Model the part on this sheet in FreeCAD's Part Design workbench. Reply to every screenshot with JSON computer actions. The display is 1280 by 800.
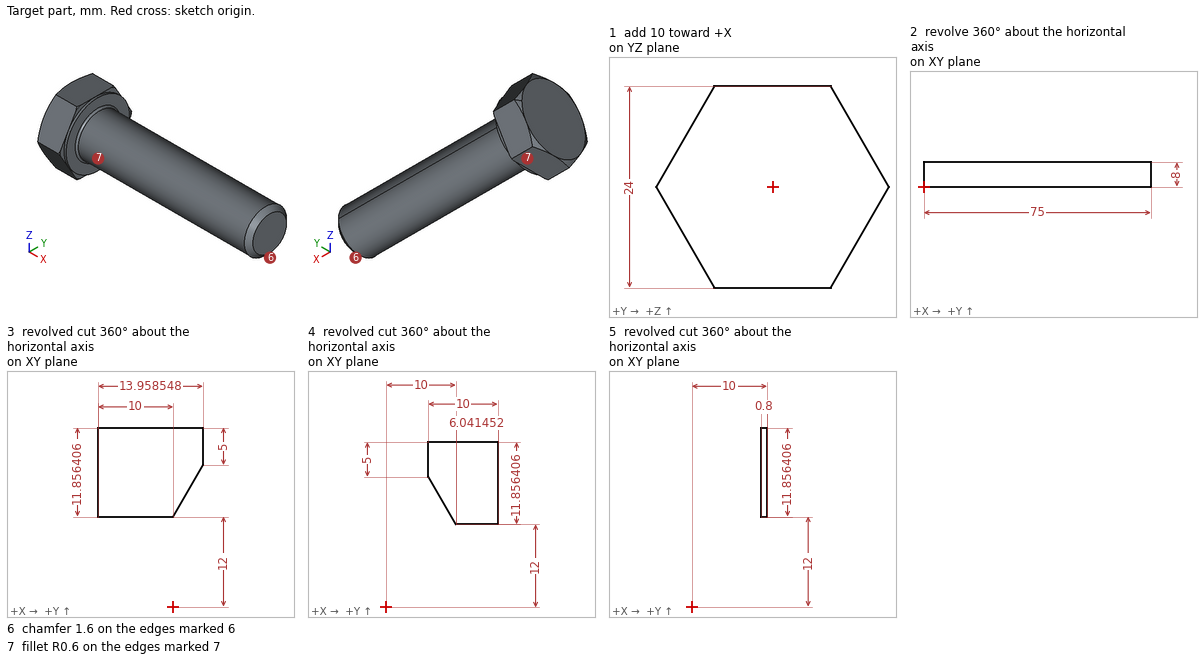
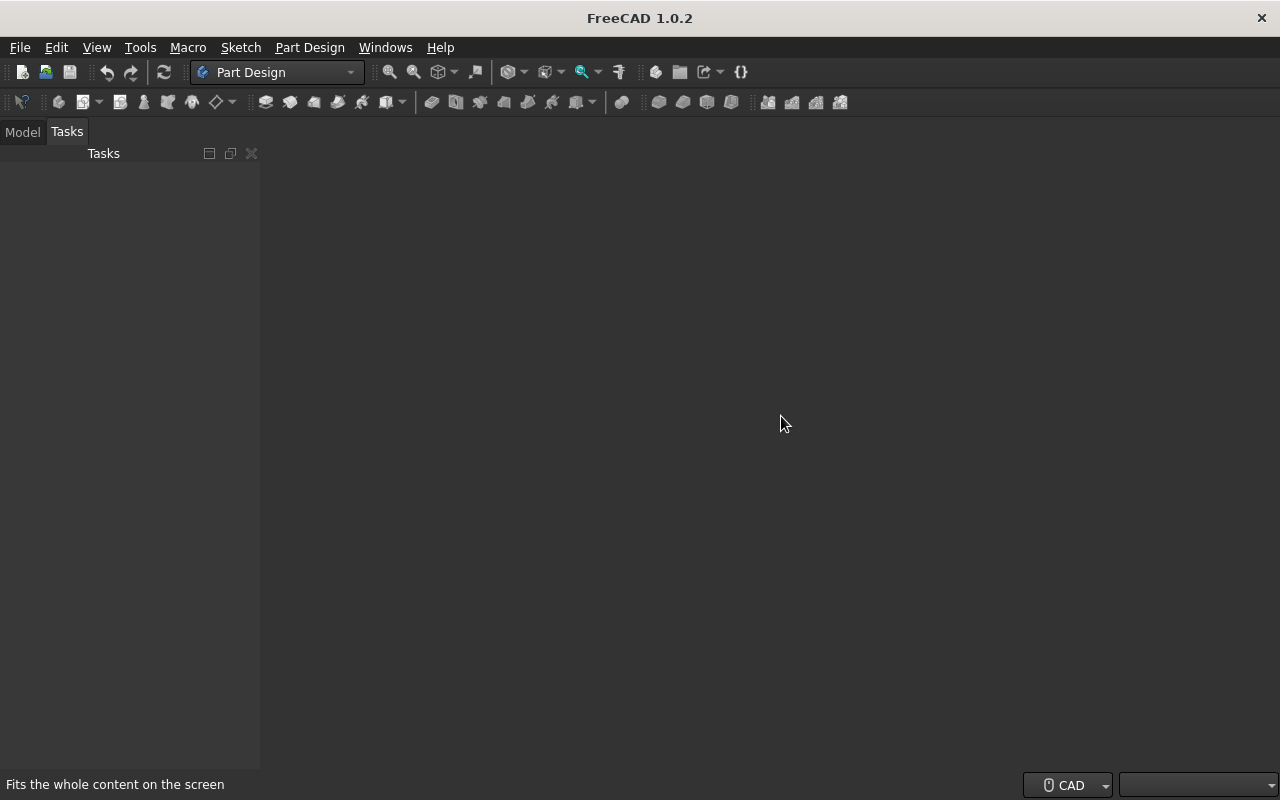
{"action": "left_click", "coordinate": [22, 72]}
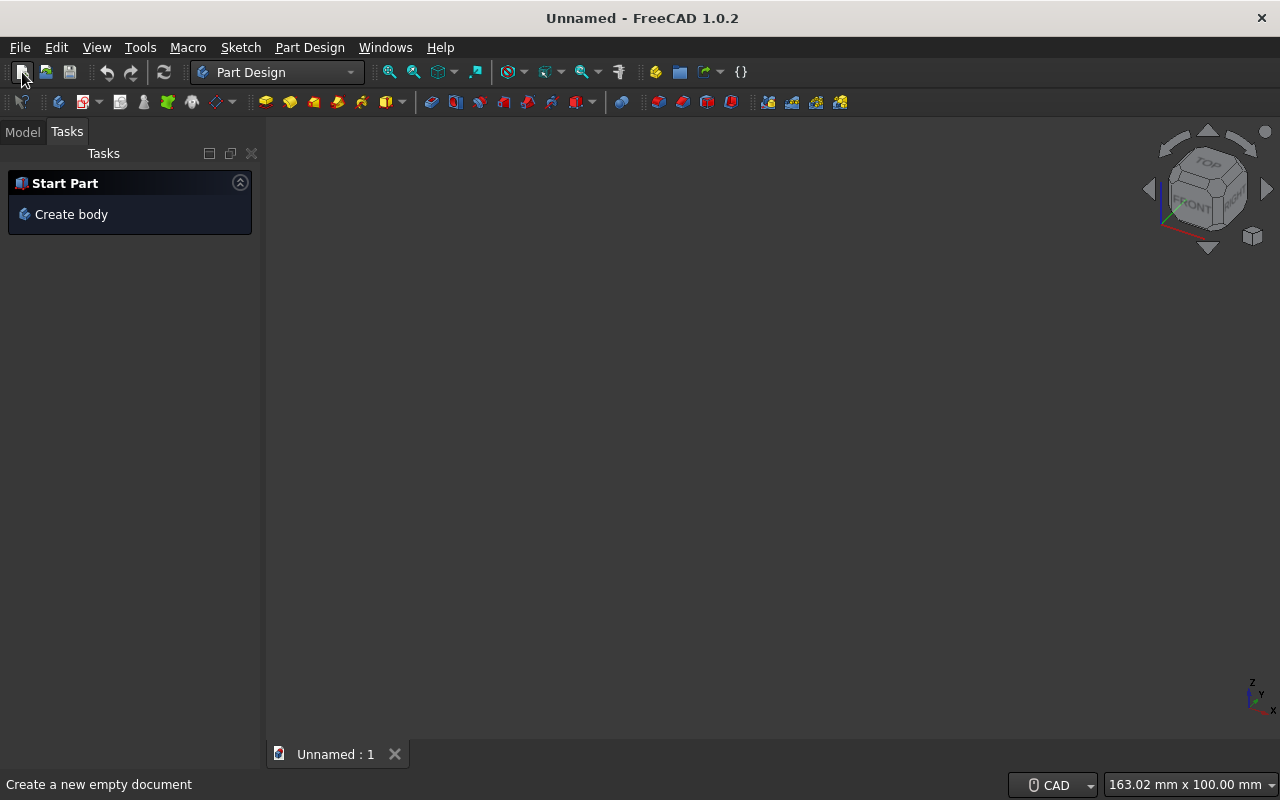
{"action": "left_click", "coordinate": [84, 102]}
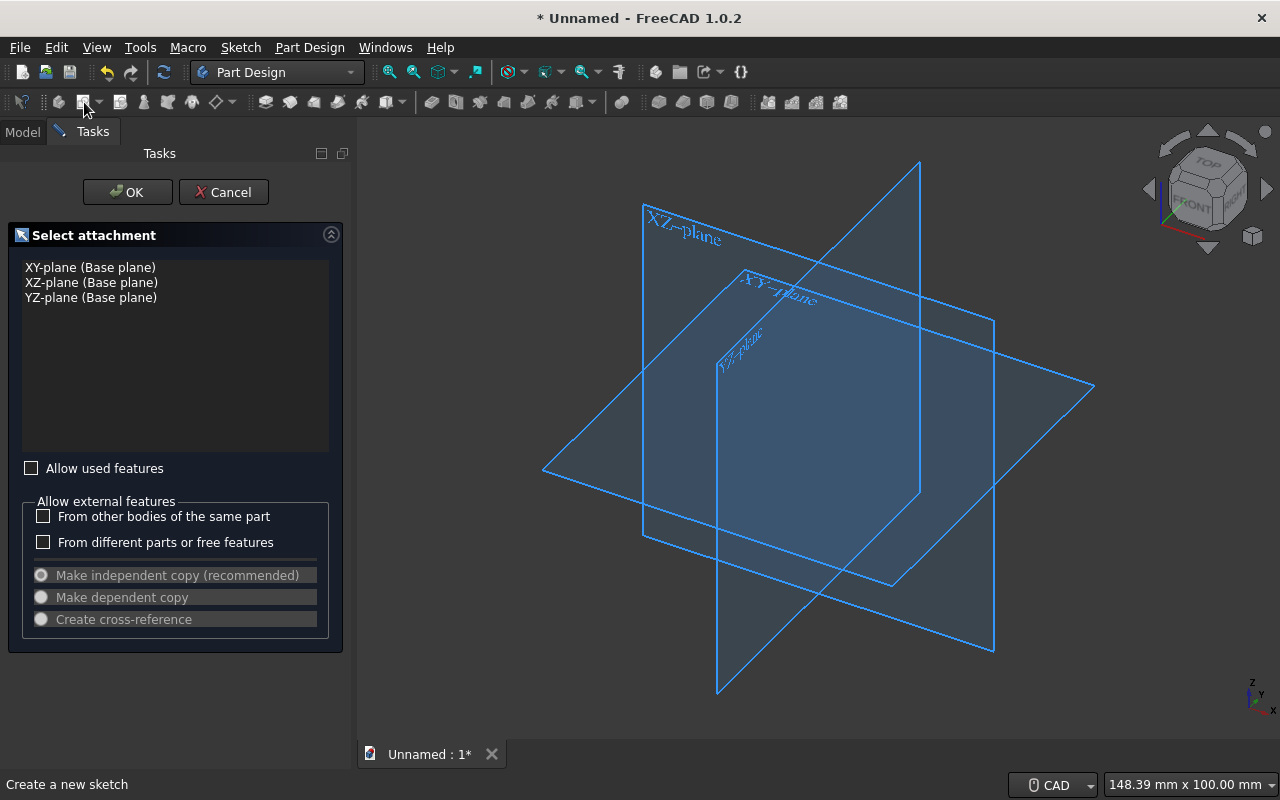
{"action": "left_click", "coordinate": [82, 298]}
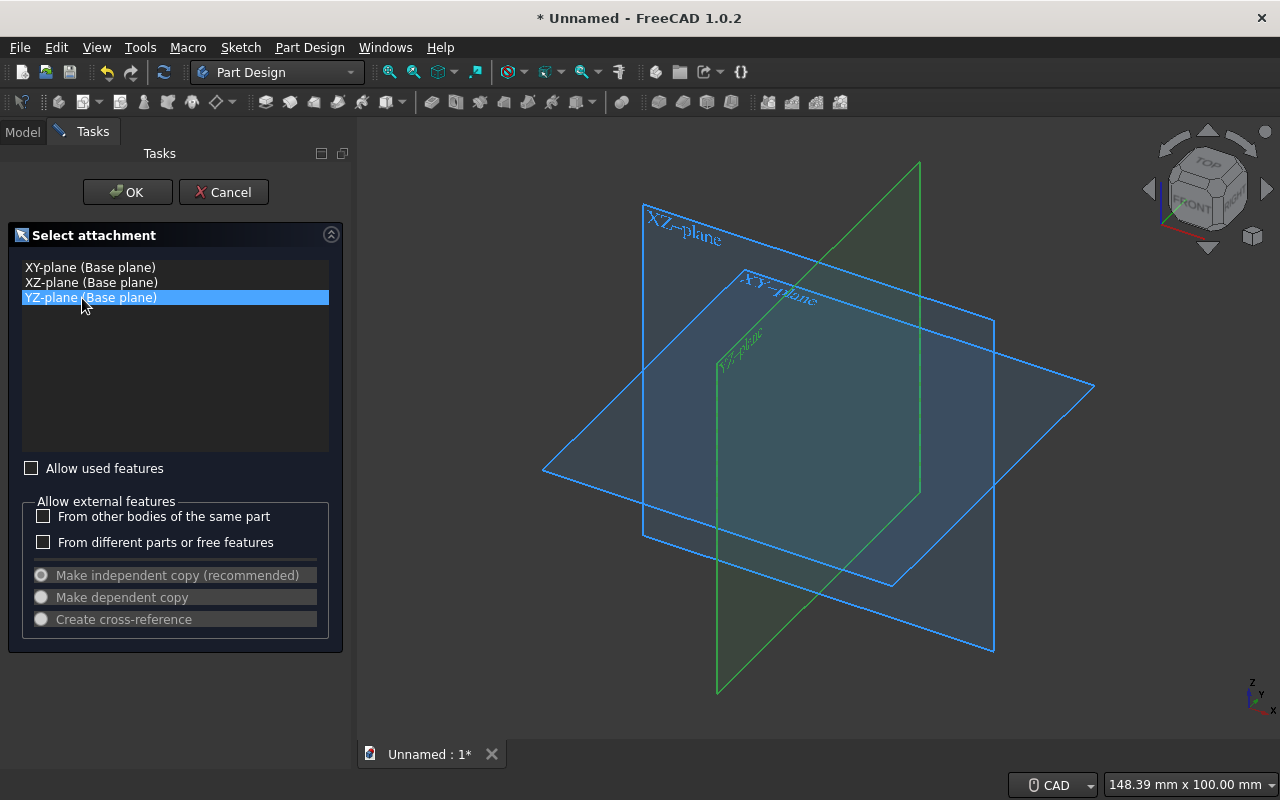
{"action": "left_click", "coordinate": [128, 192]}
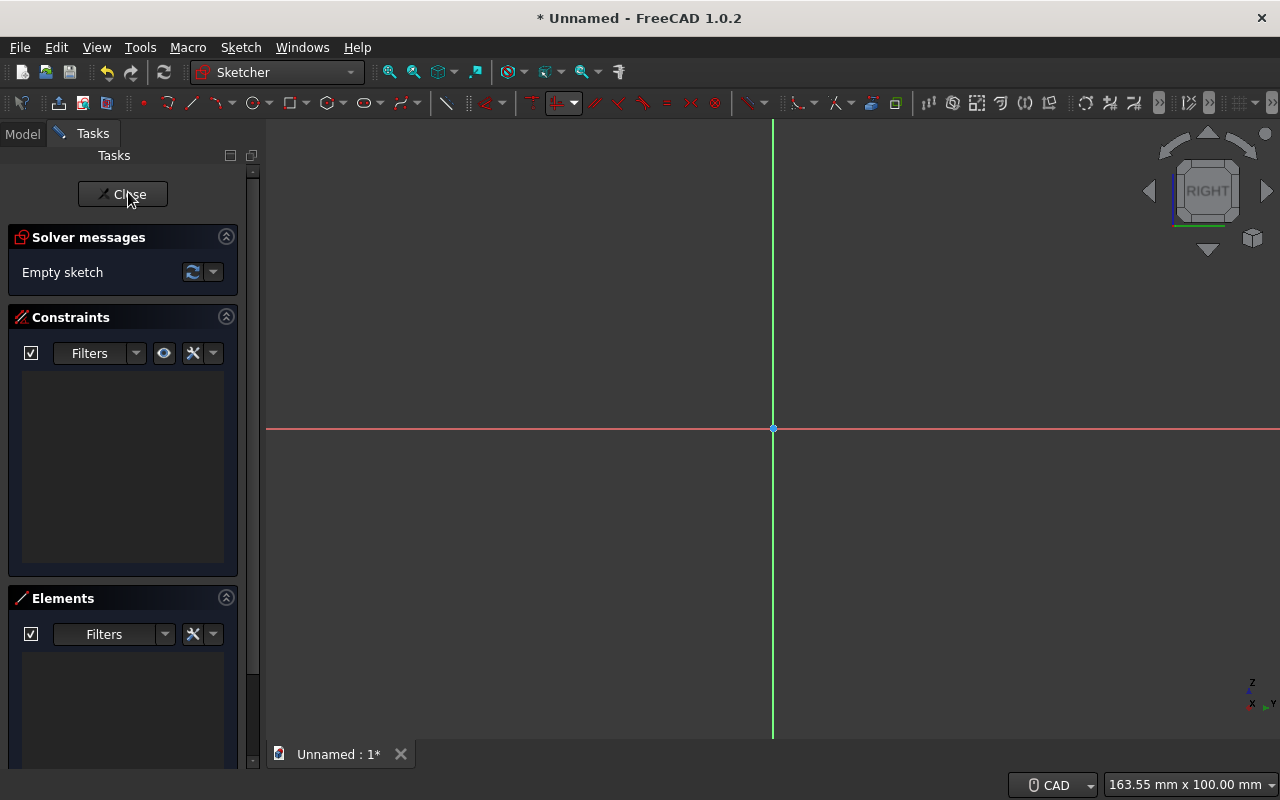
{"action": "scroll", "coordinate": [813, 429], "scroll_direction": "up", "scroll_amount": 5}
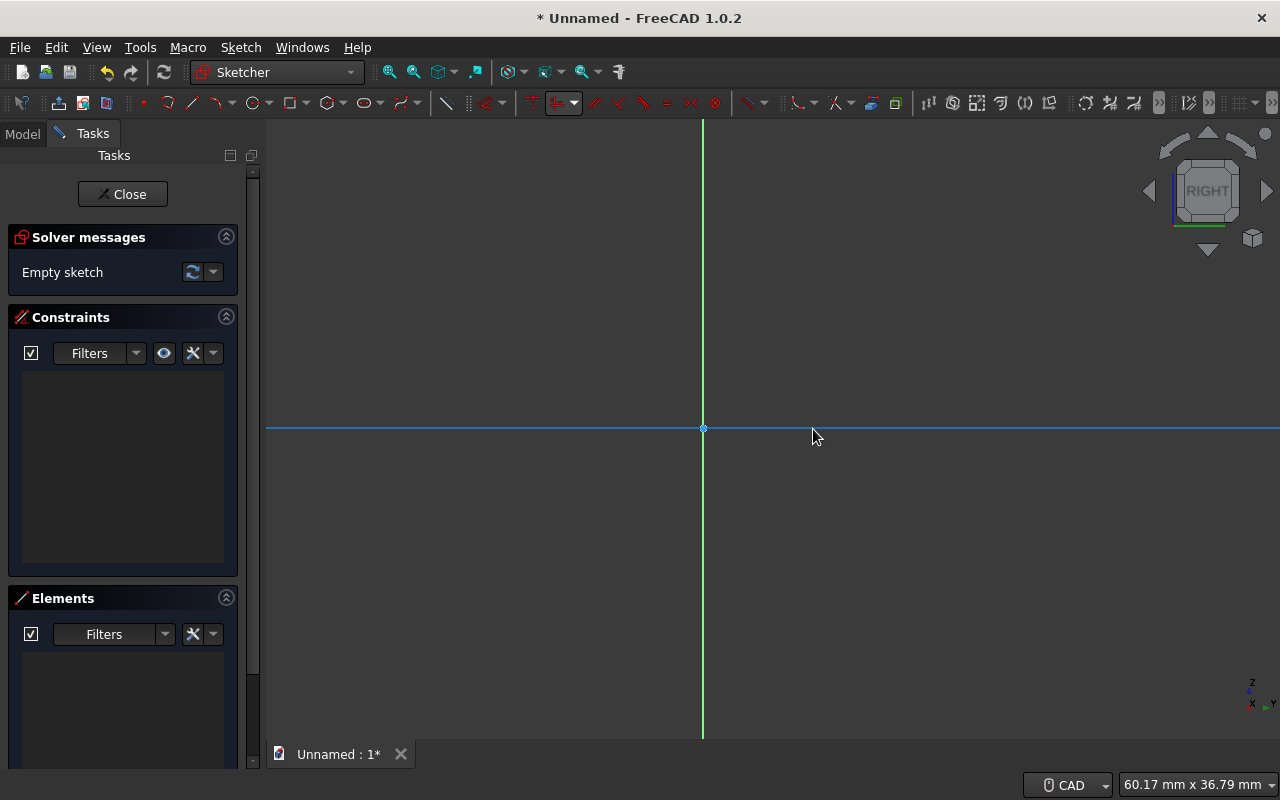
{"action": "left_click", "coordinate": [328, 104]}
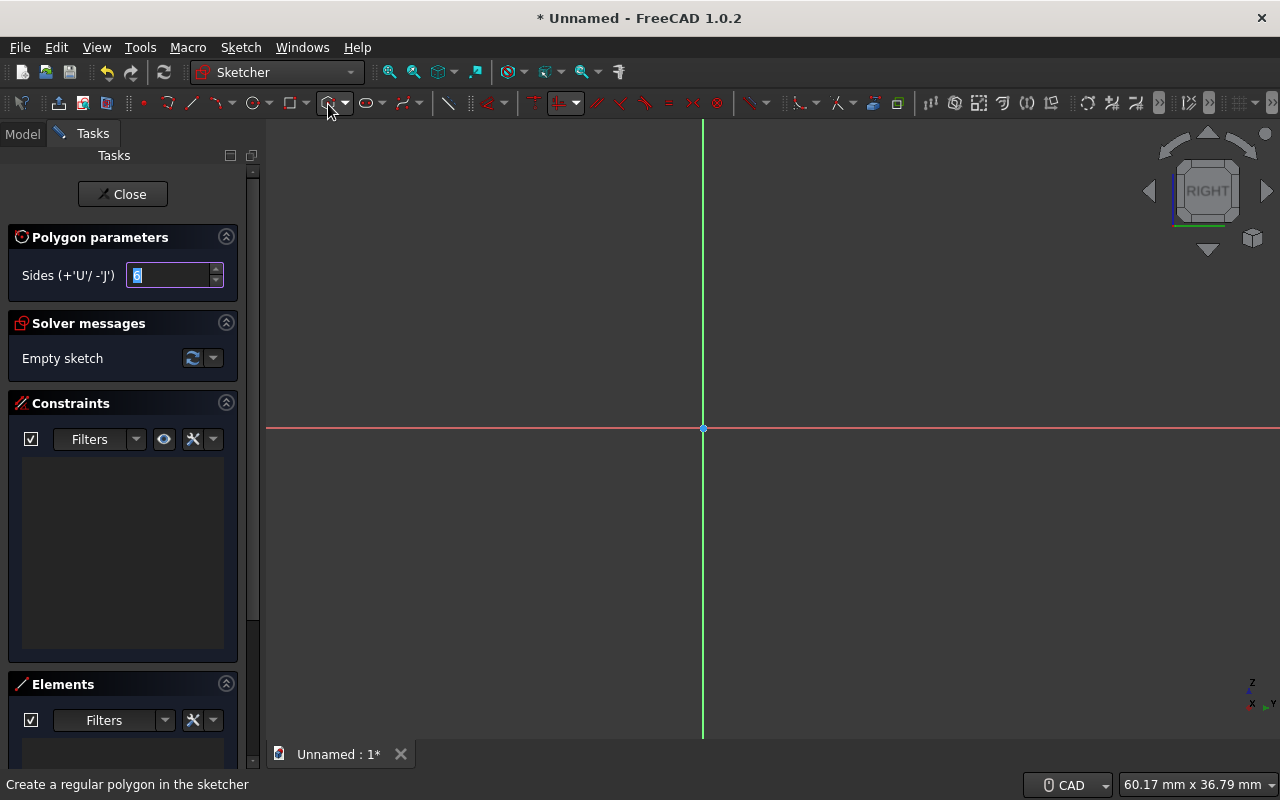
{"action": "left_click", "coordinate": [703, 428]}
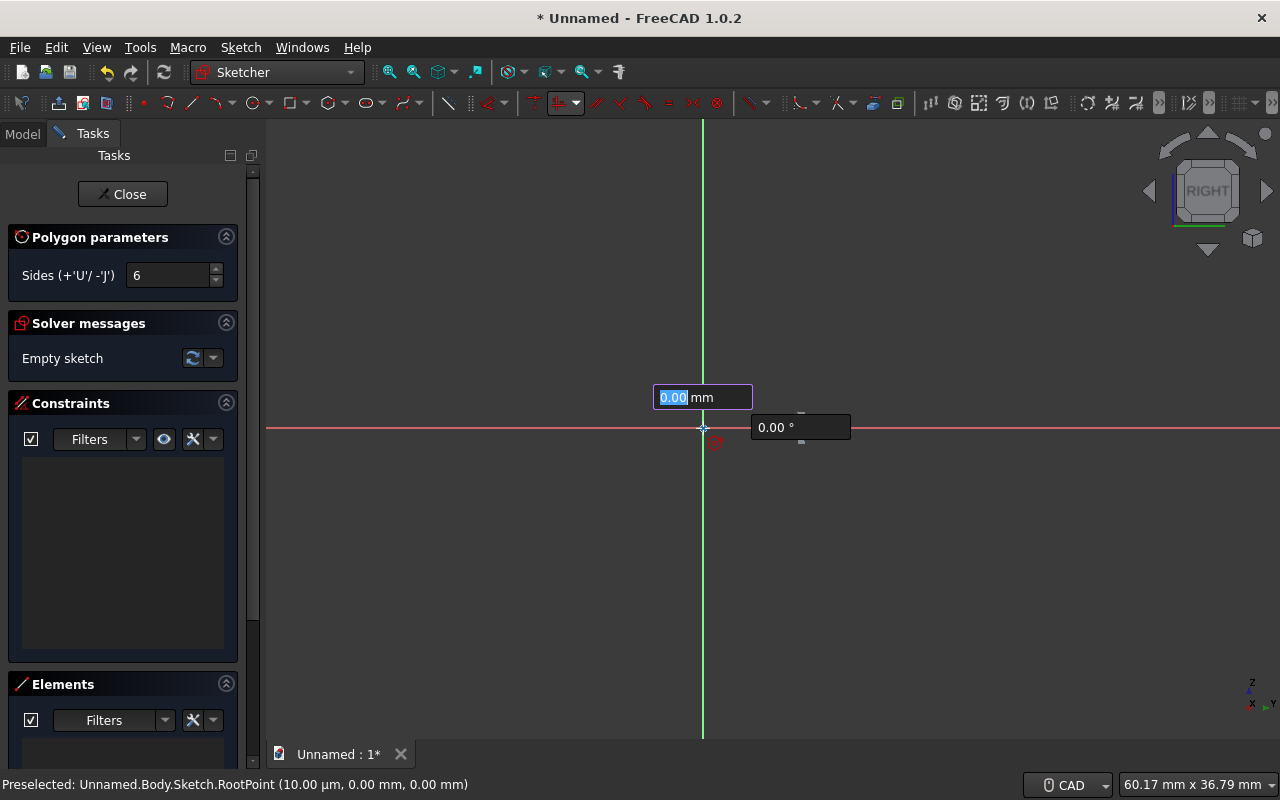
{"action": "left_click", "coordinate": [937, 428]}
{"action": "right_click", "coordinate": [937, 428]}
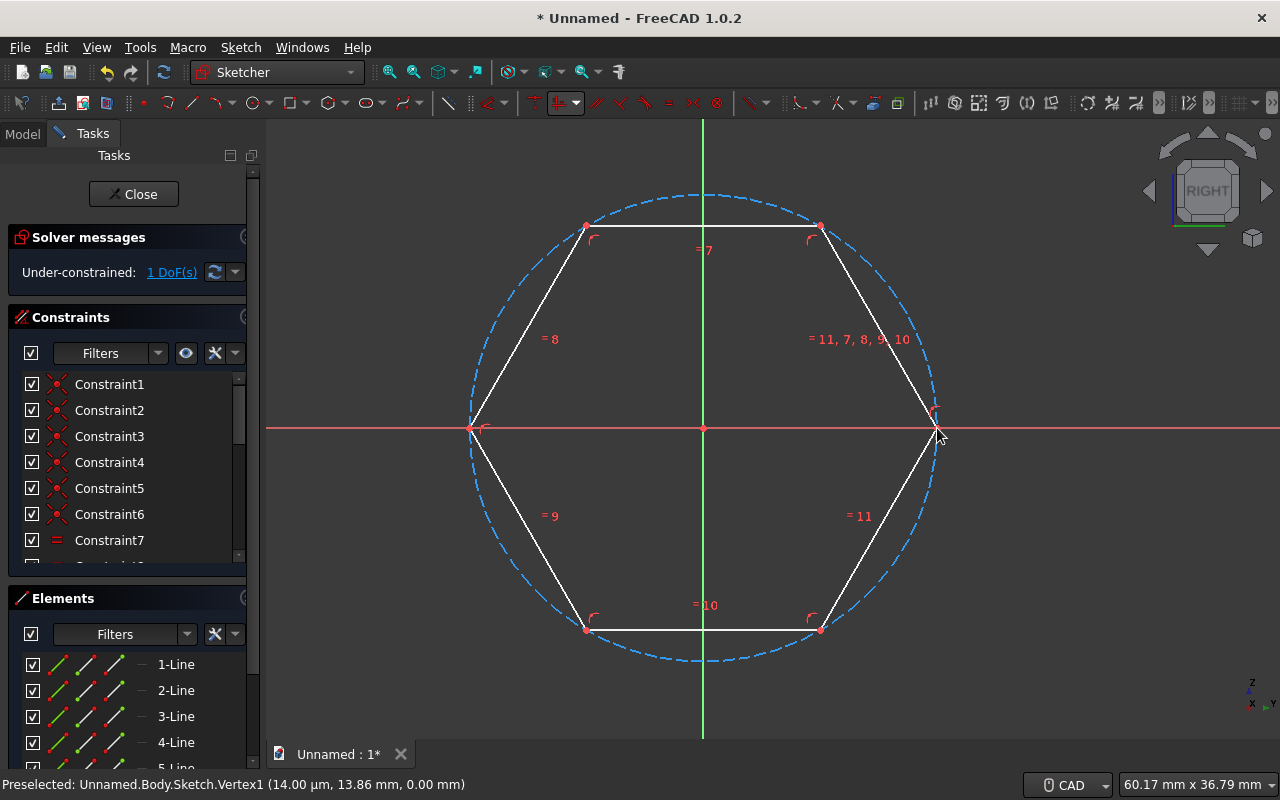
{"action": "left_click", "coordinate": [488, 104]}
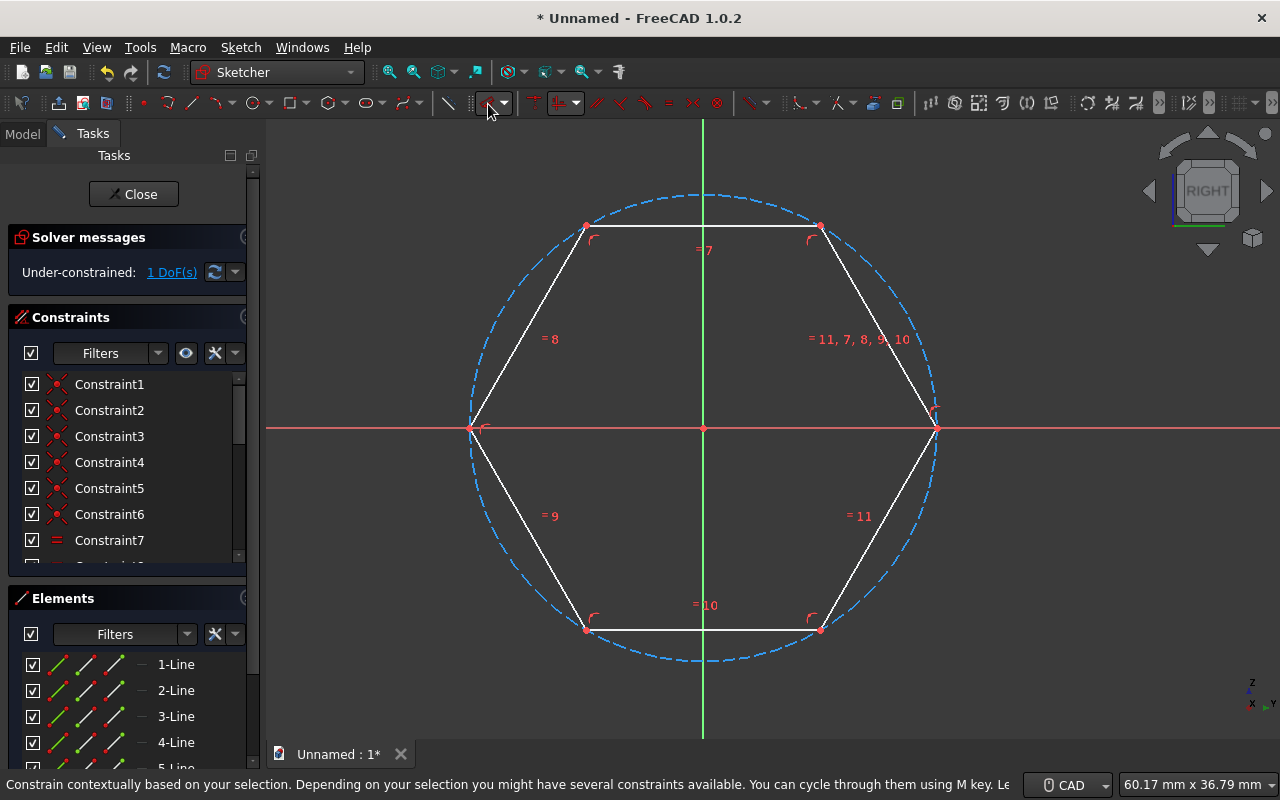
{"action": "left_click", "coordinate": [587, 630]}